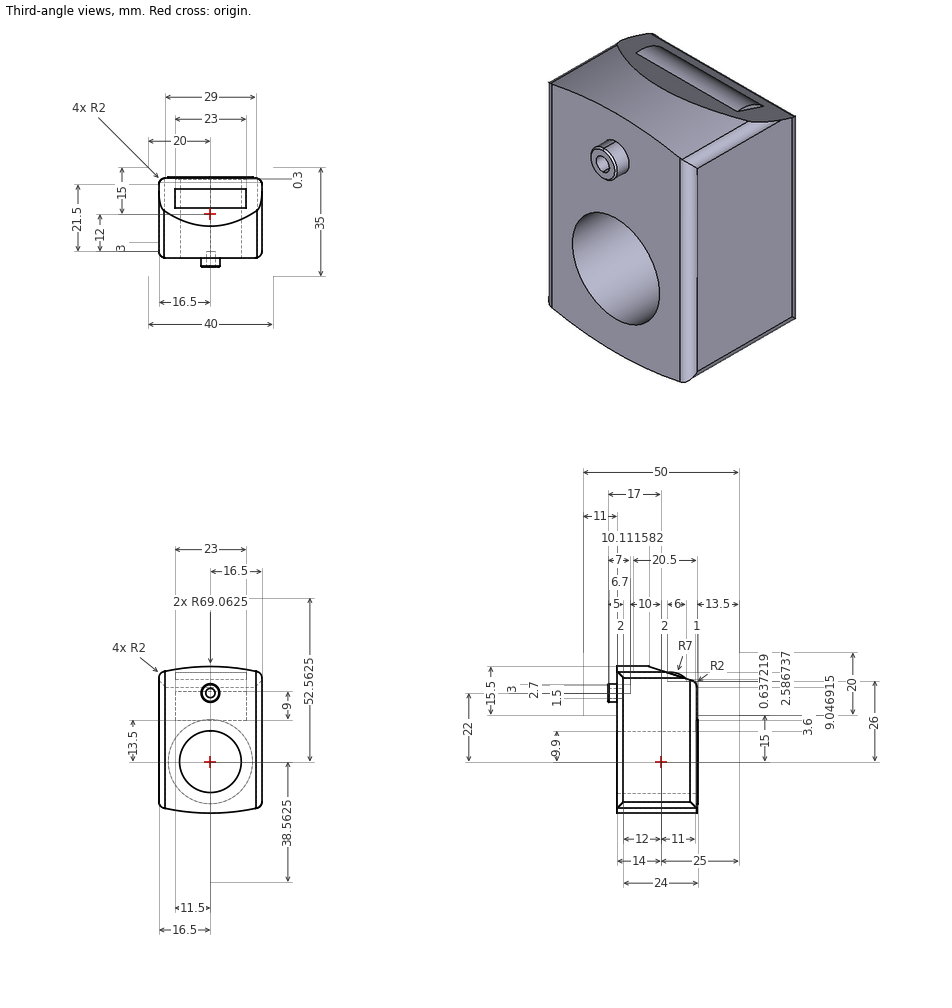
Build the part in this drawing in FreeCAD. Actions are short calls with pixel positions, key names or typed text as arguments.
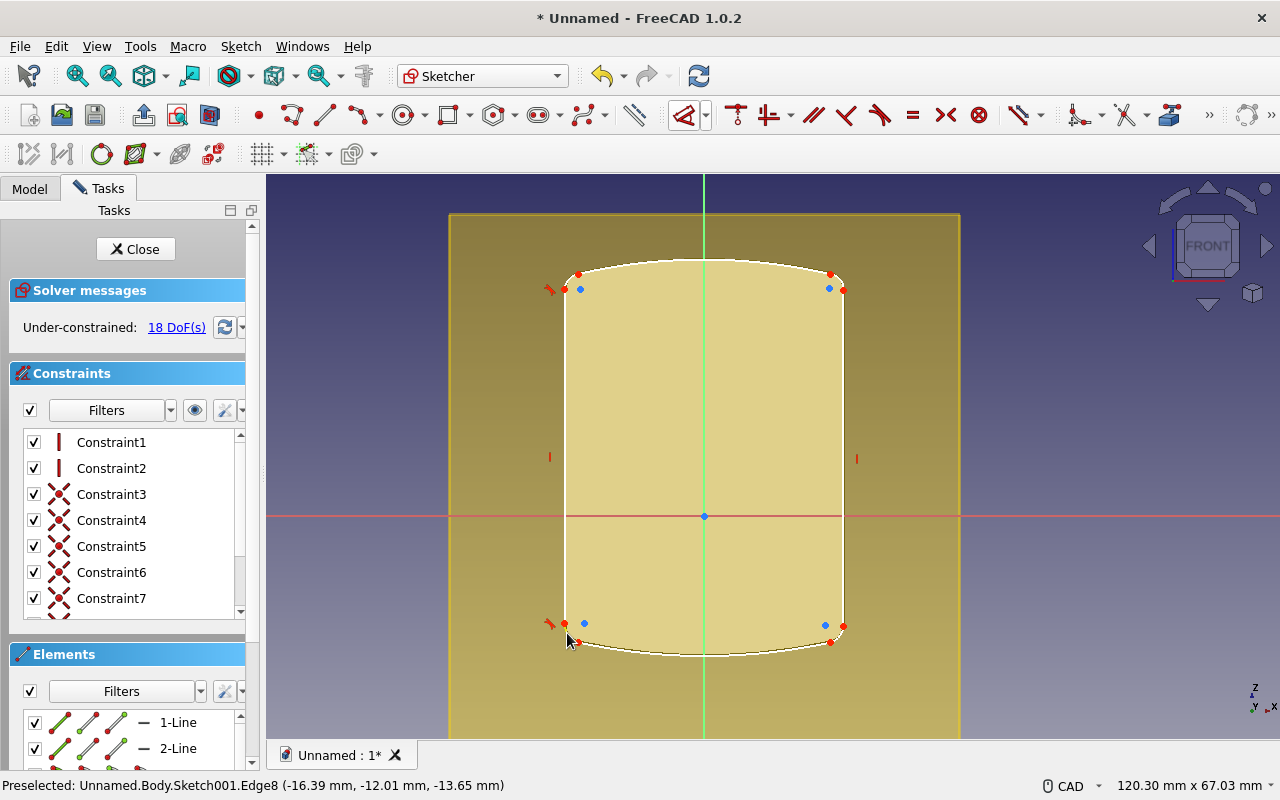
click(843, 391)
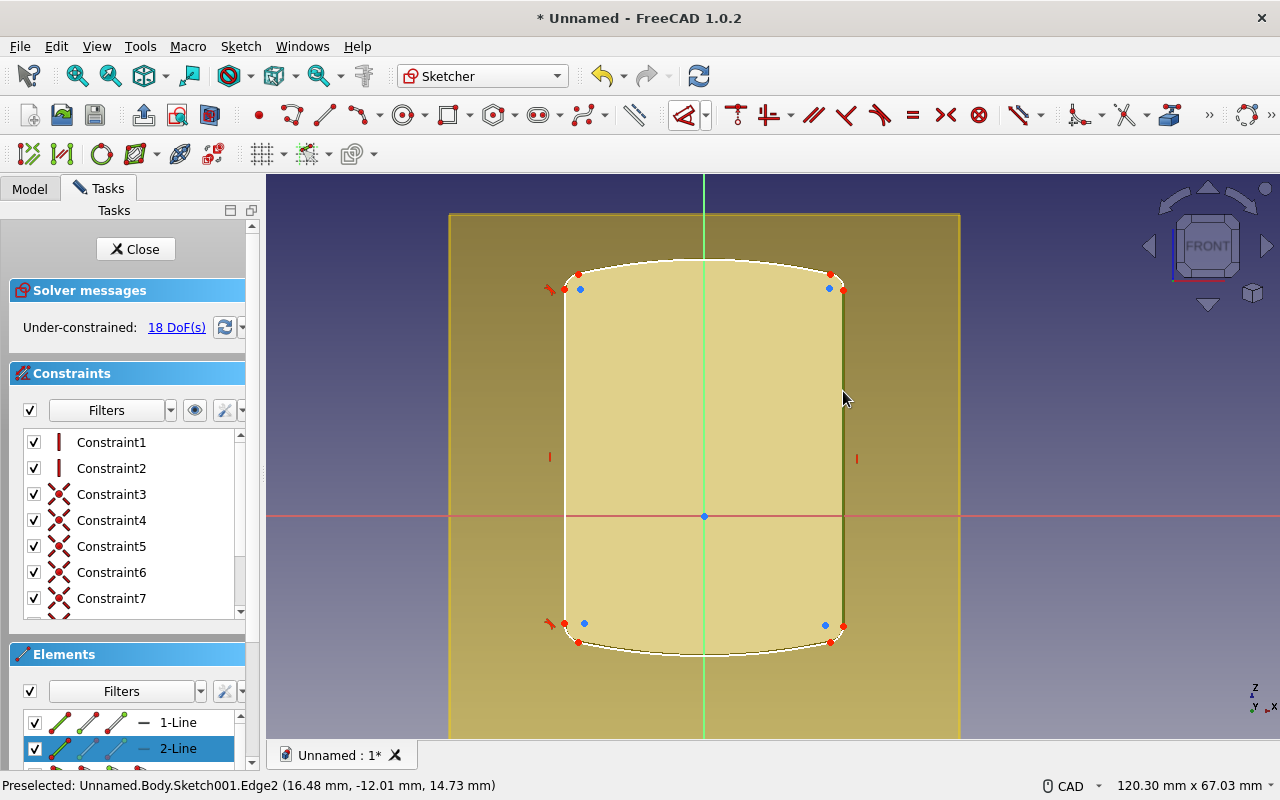
scroll(840, 279, up, 2)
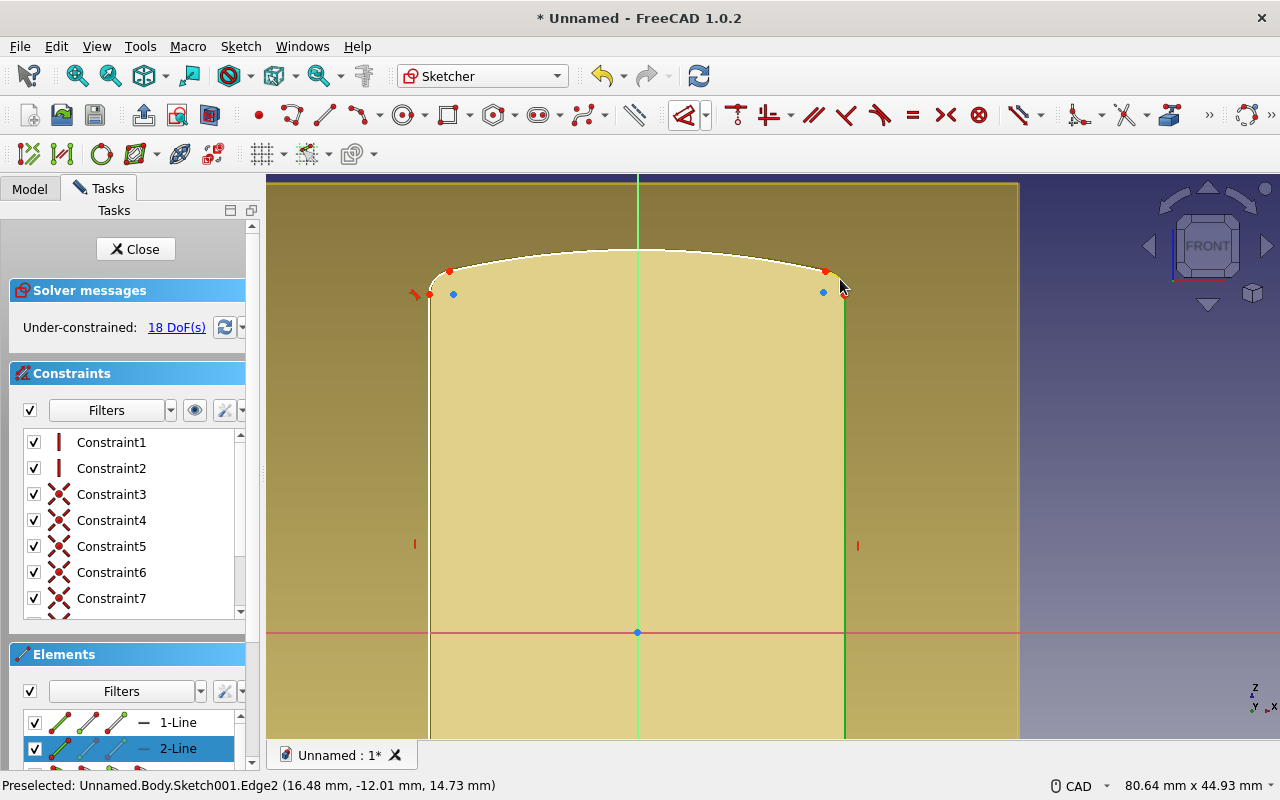
click(840, 279)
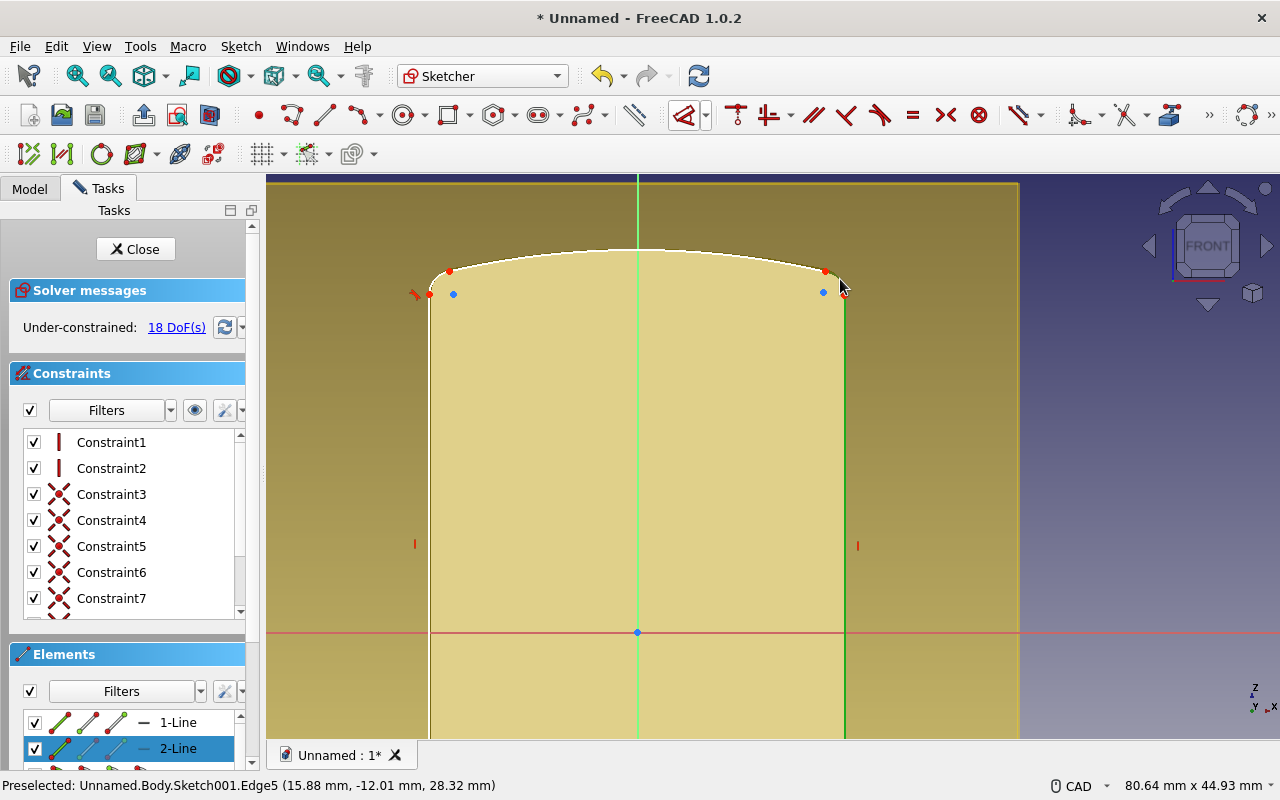
click(880, 116)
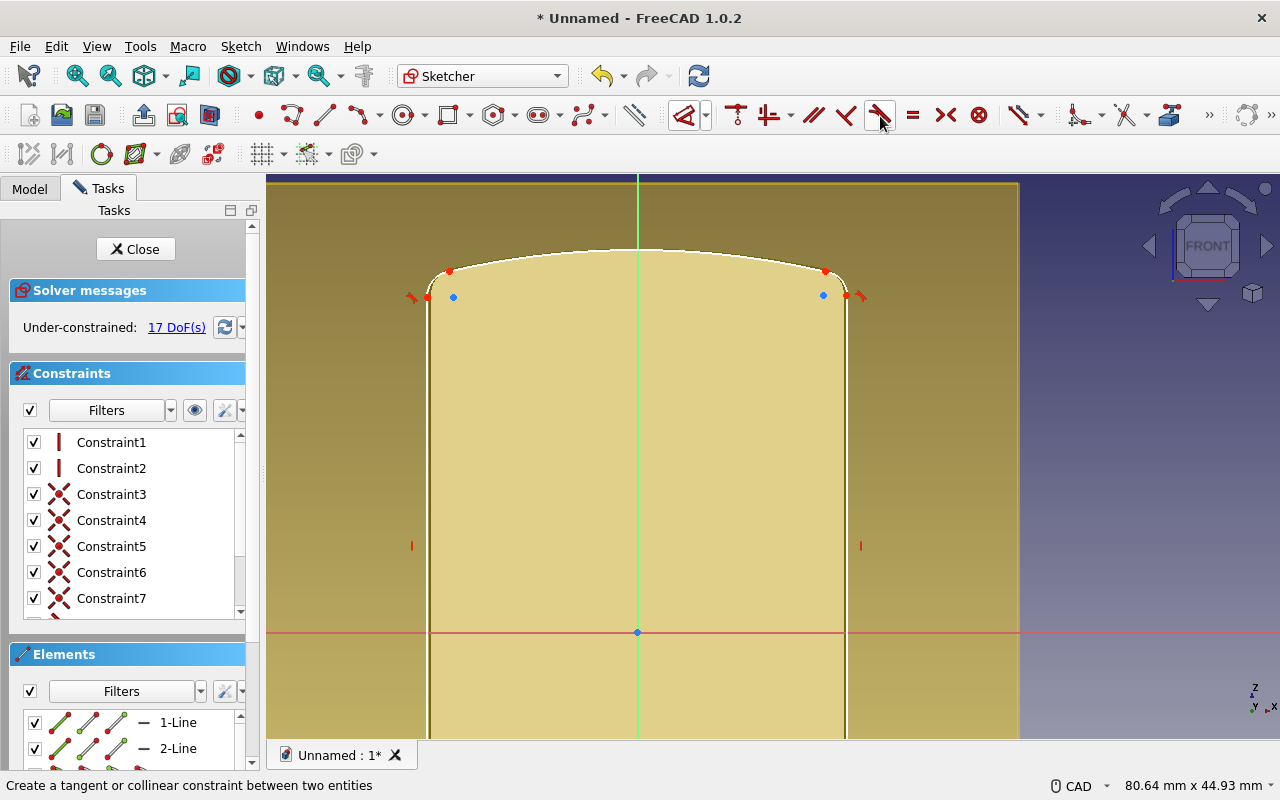
click(847, 446)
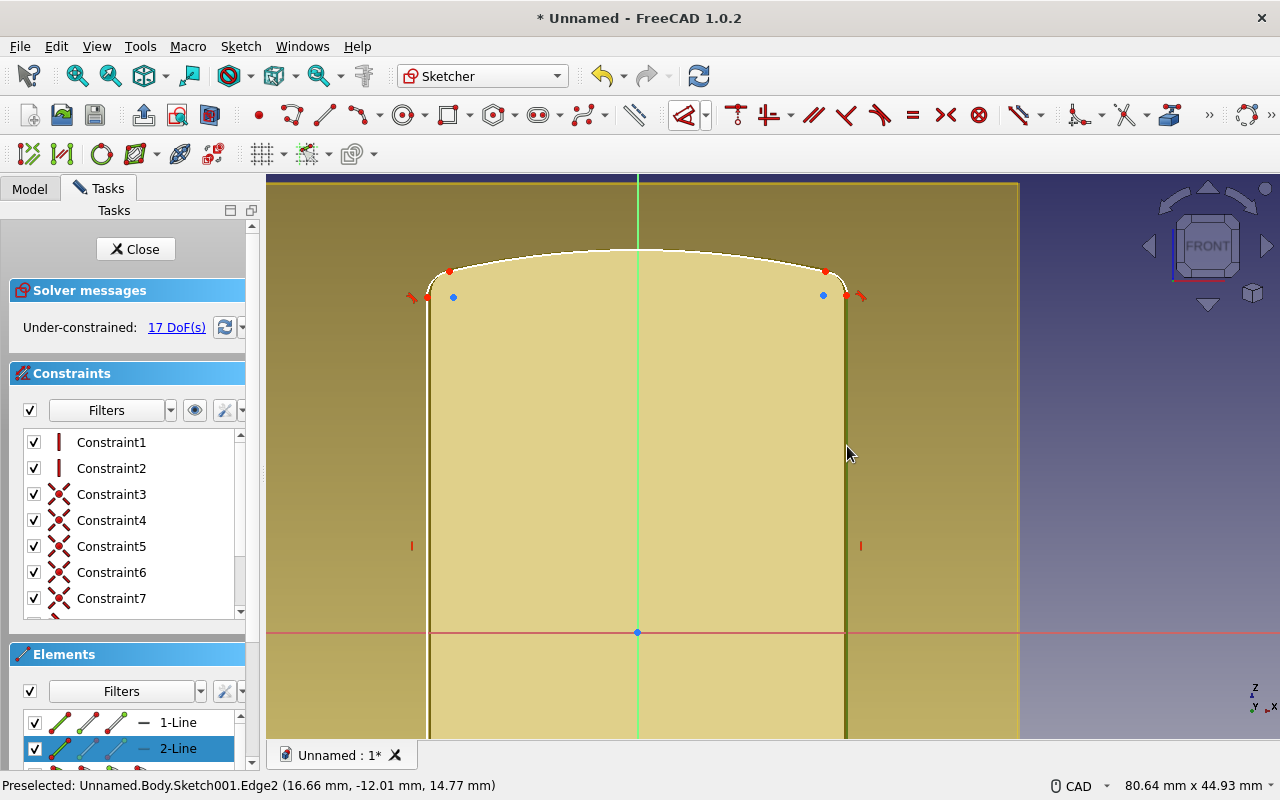
scroll(841, 277, down, 2)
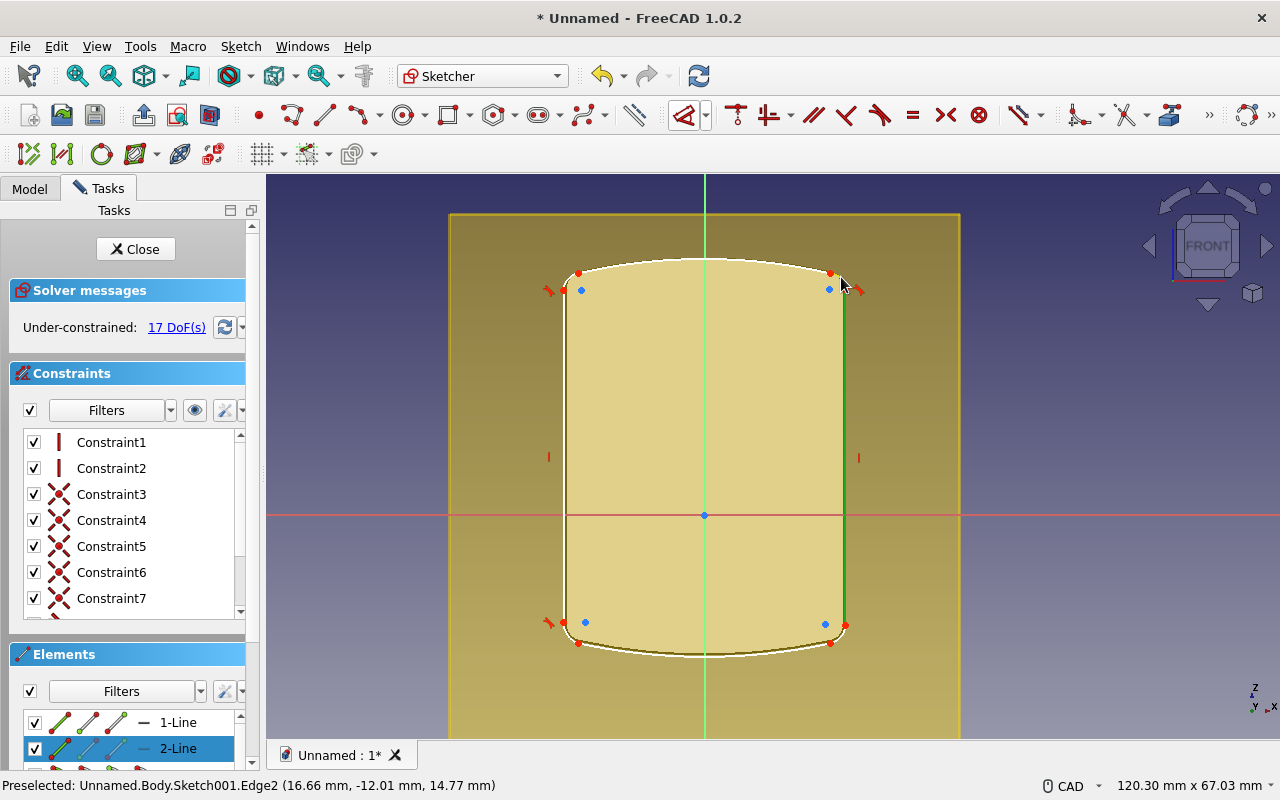
scroll(837, 640, up, 4)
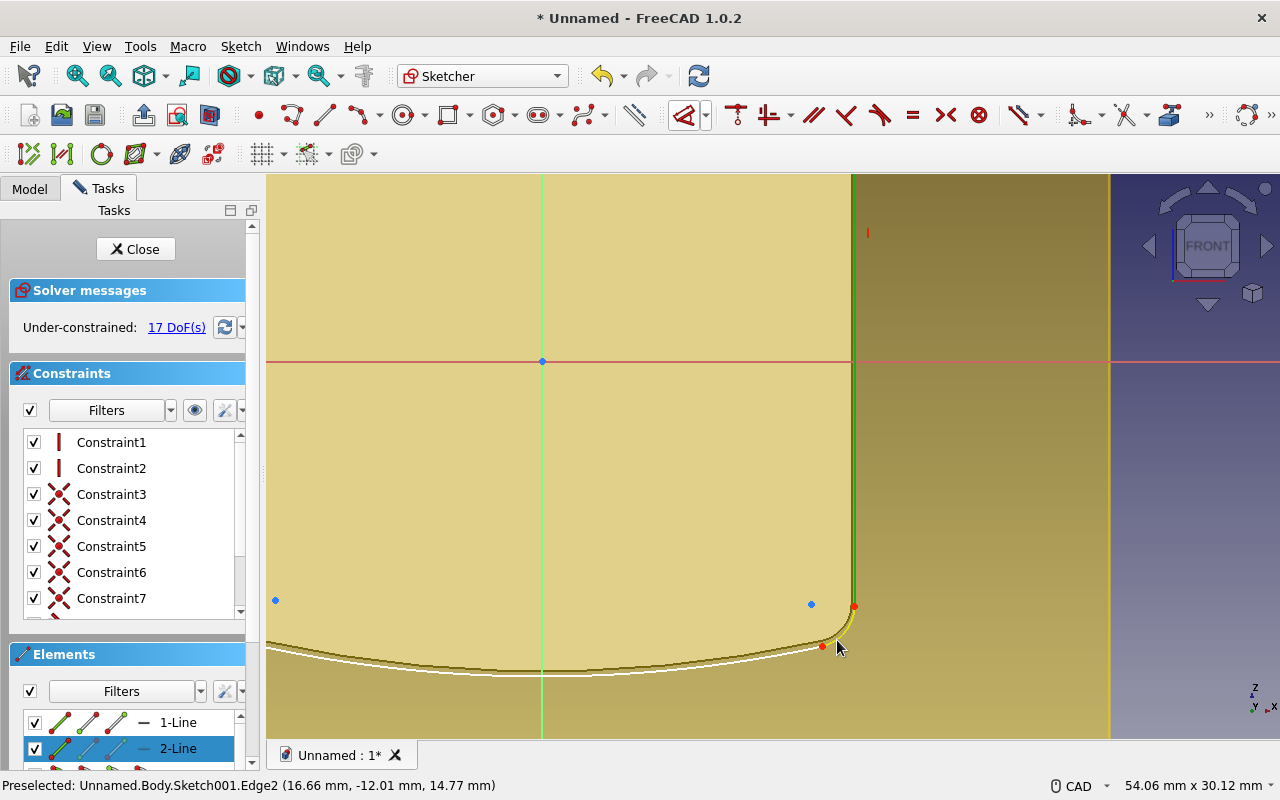
click(837, 639)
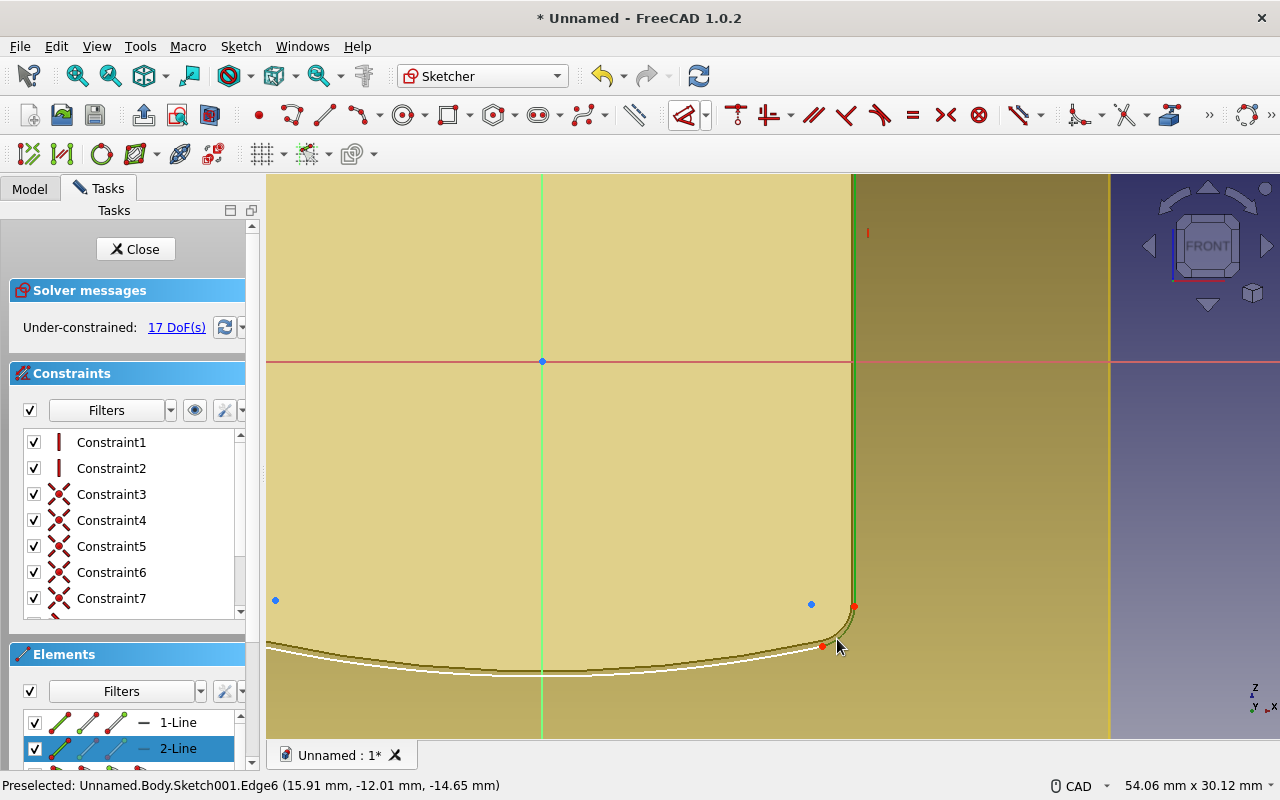
click(880, 116)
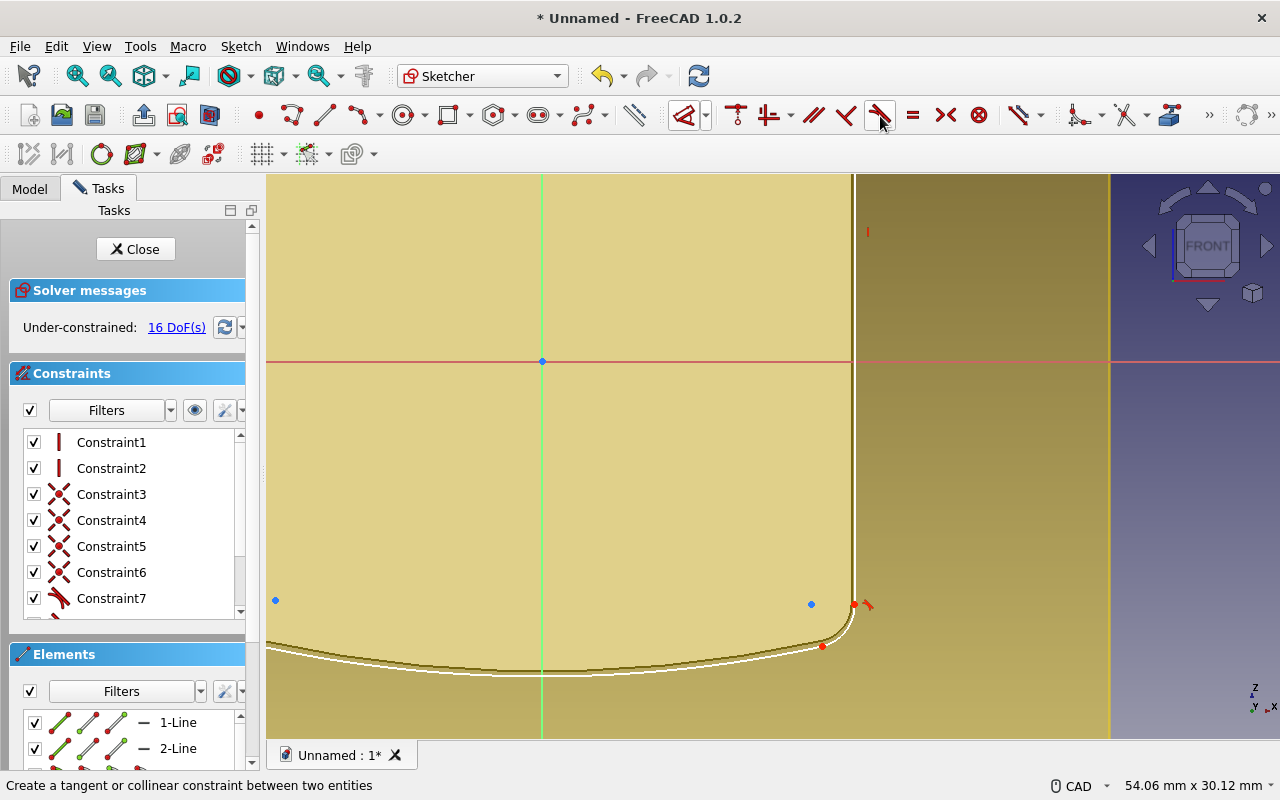
scroll(837, 641, down, 4)